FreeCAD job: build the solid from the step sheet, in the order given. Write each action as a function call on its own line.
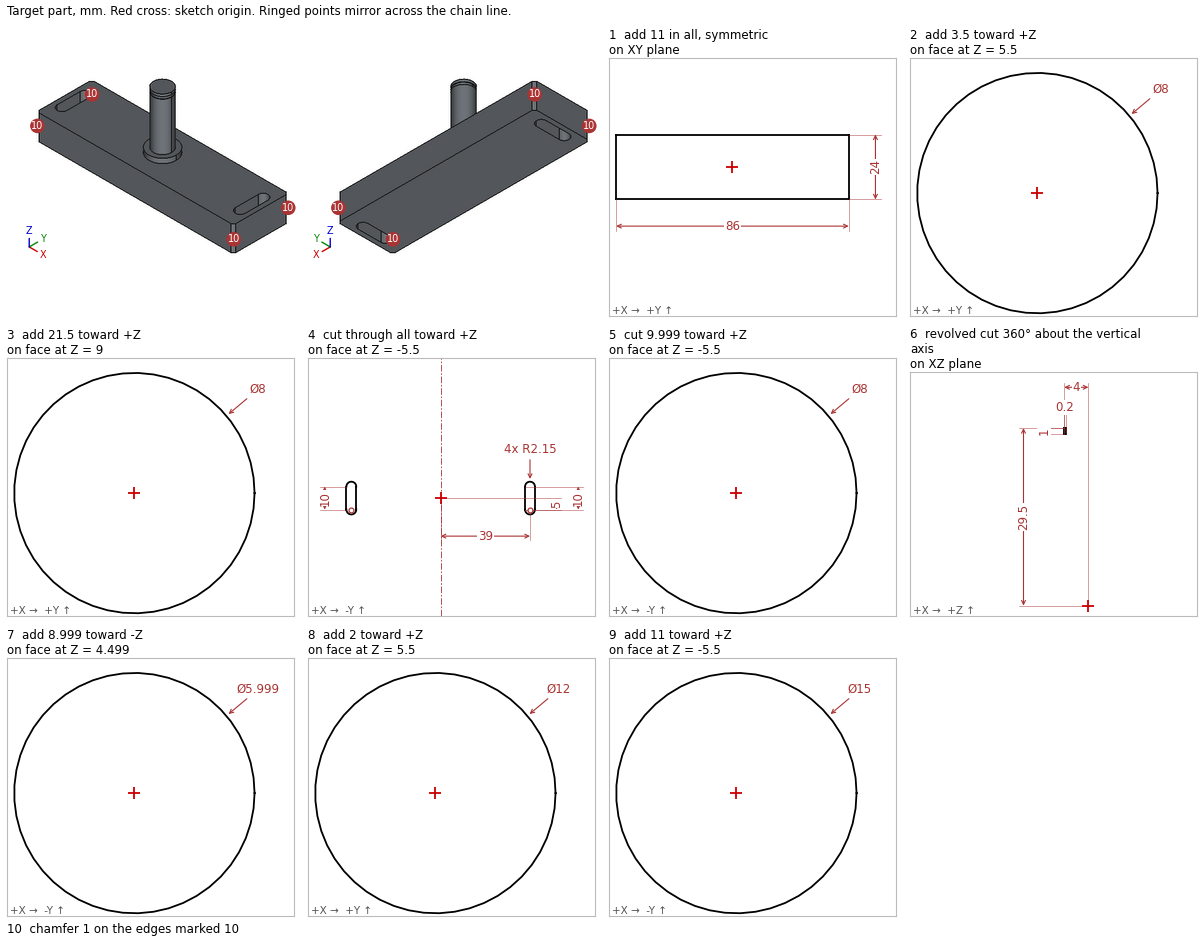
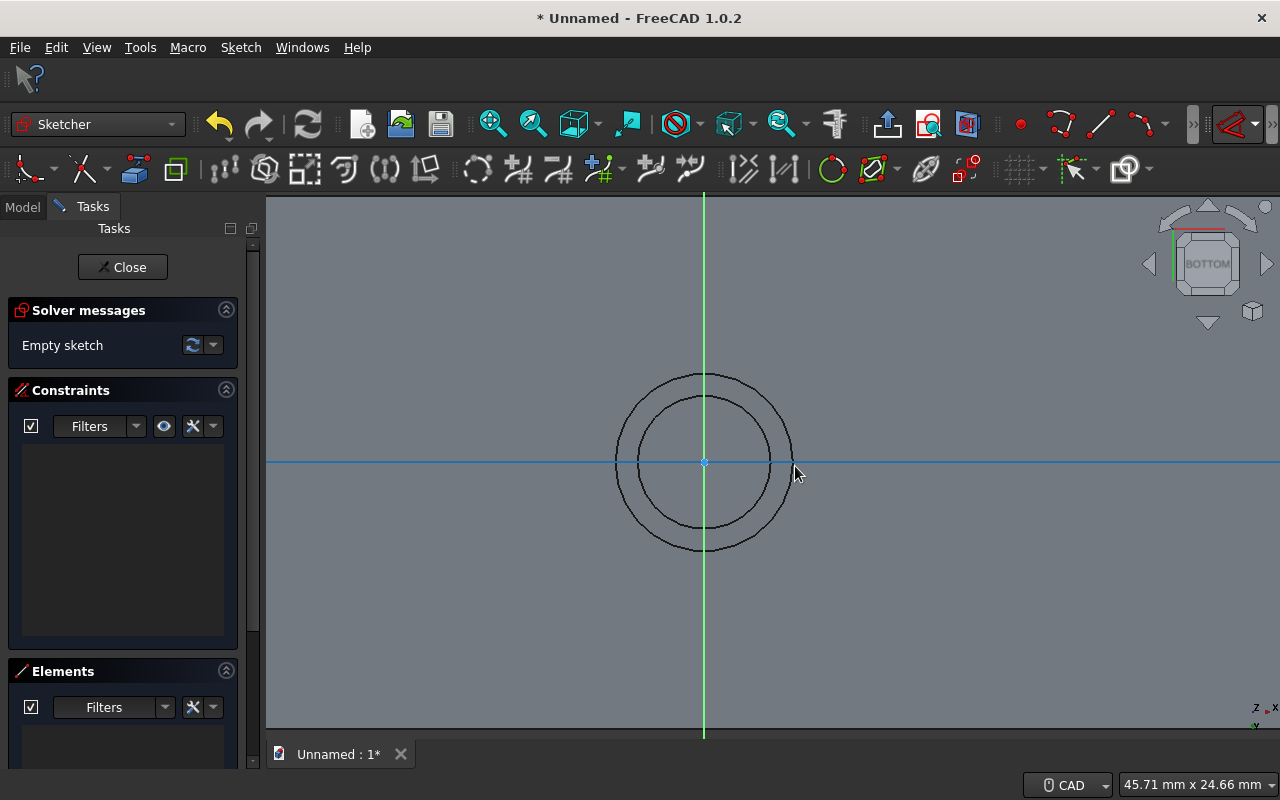
key(g)
key(c)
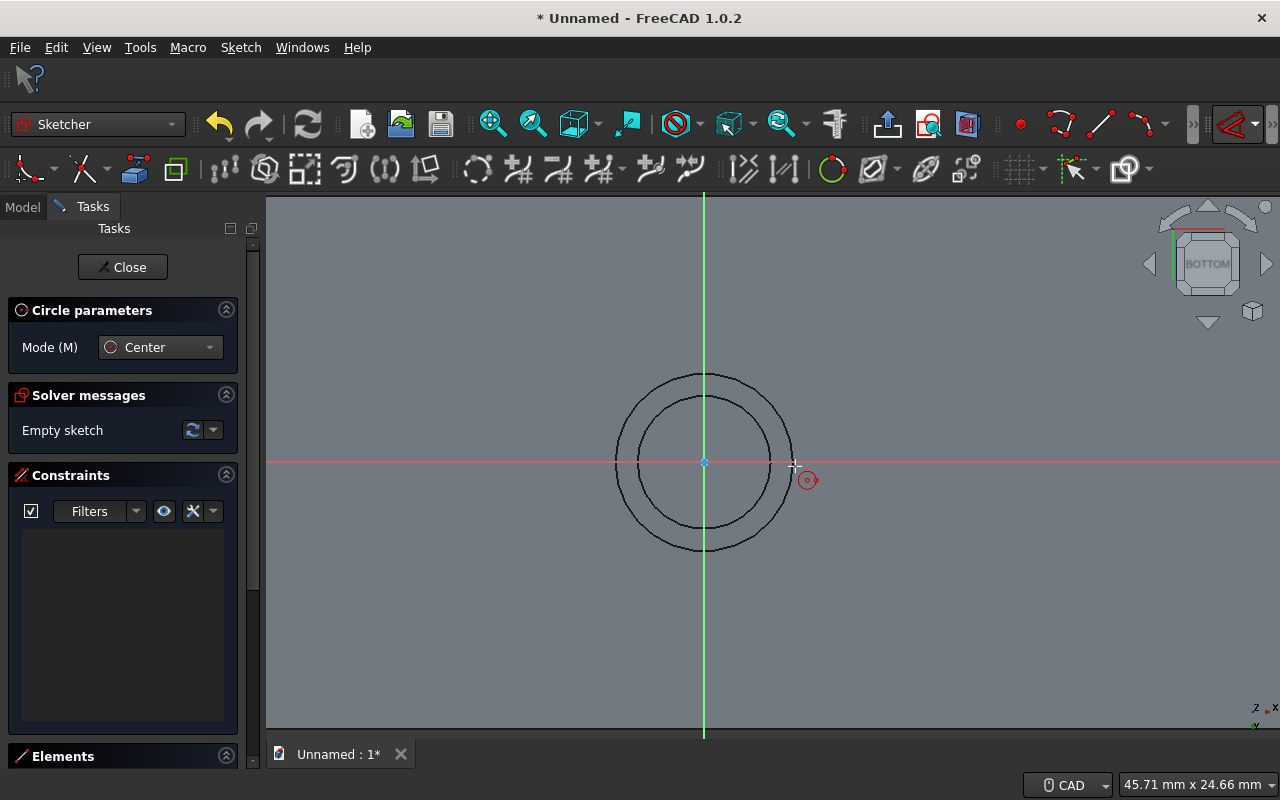
click(704, 462)
move(822, 345)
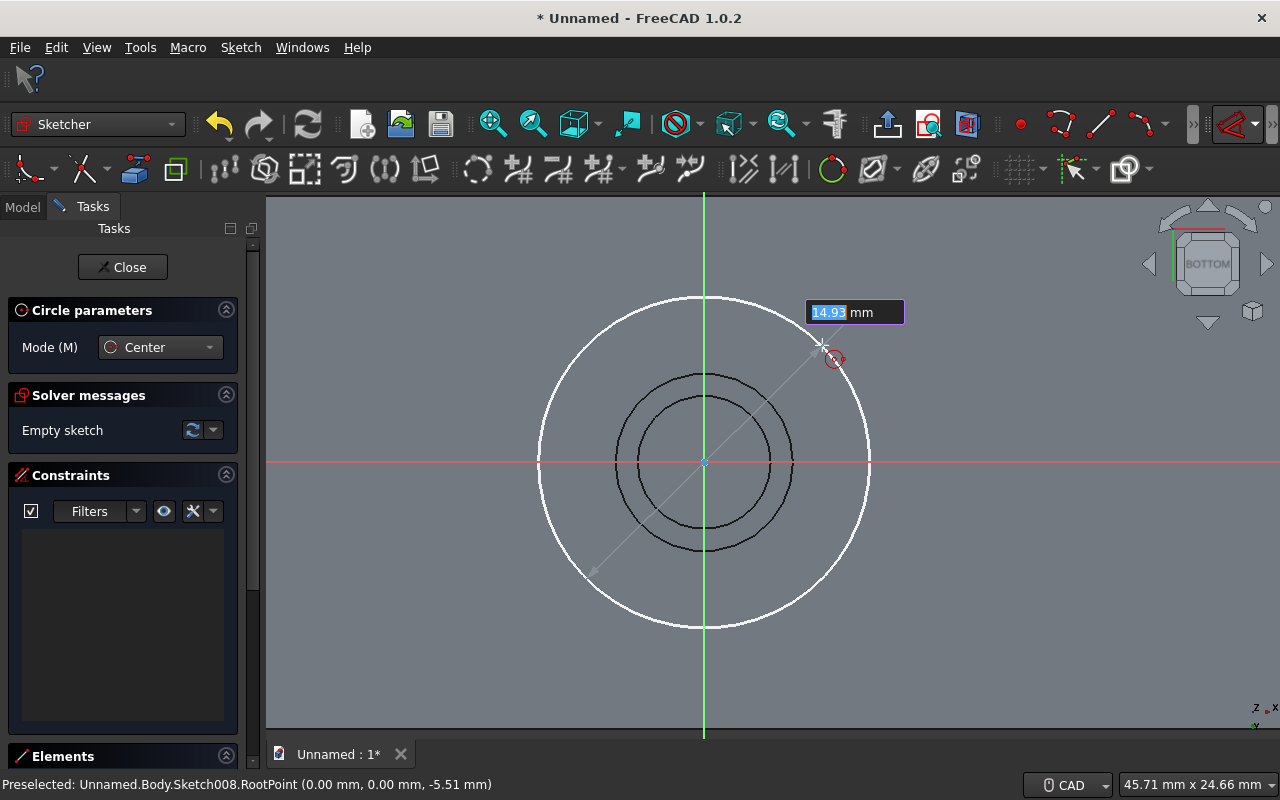
text(15)
key(Return)
key(Escape)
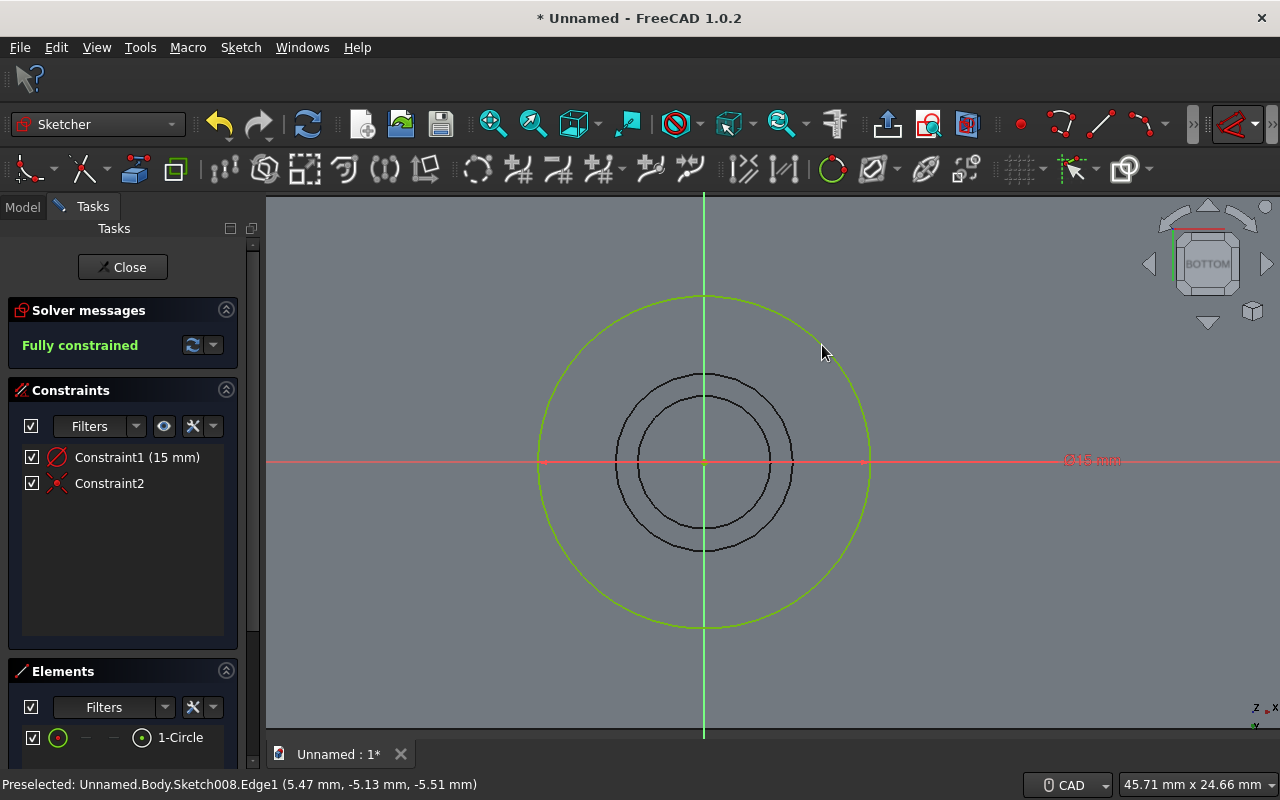
click(123, 267)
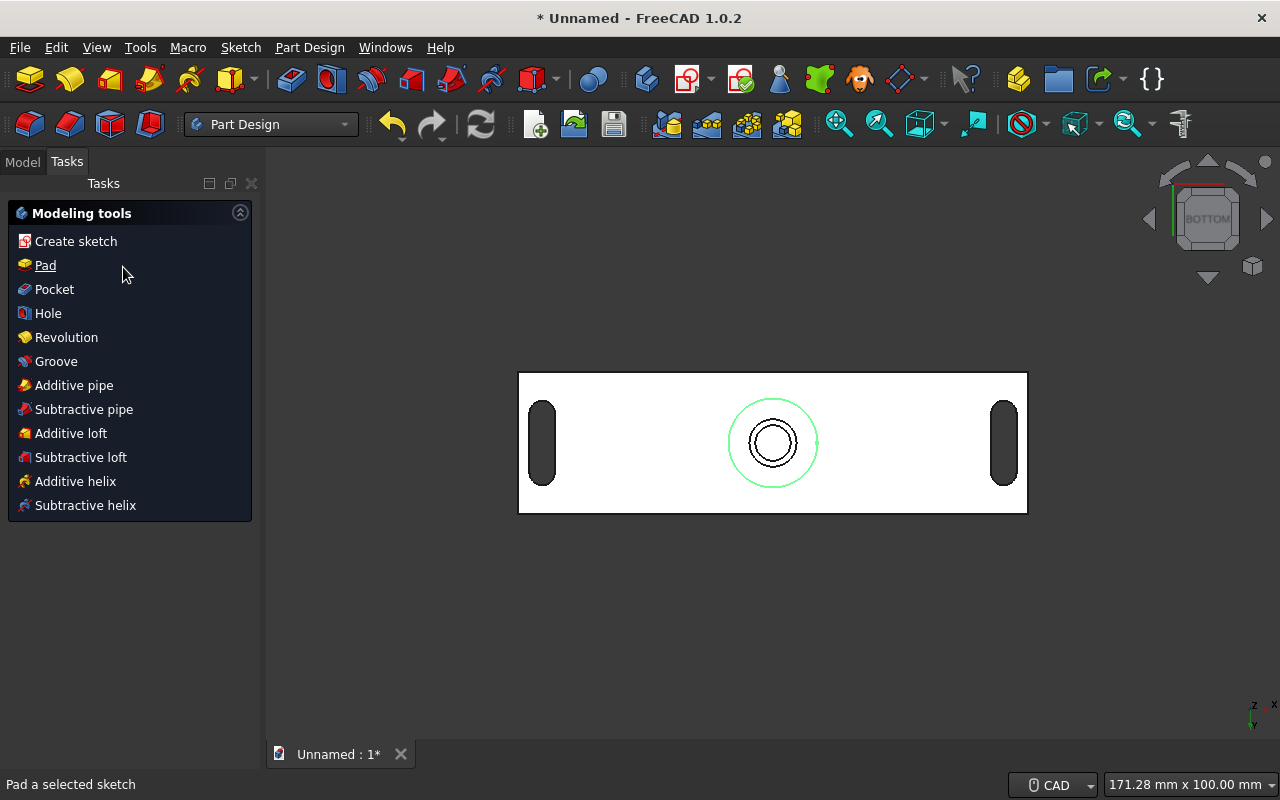
click(30, 80)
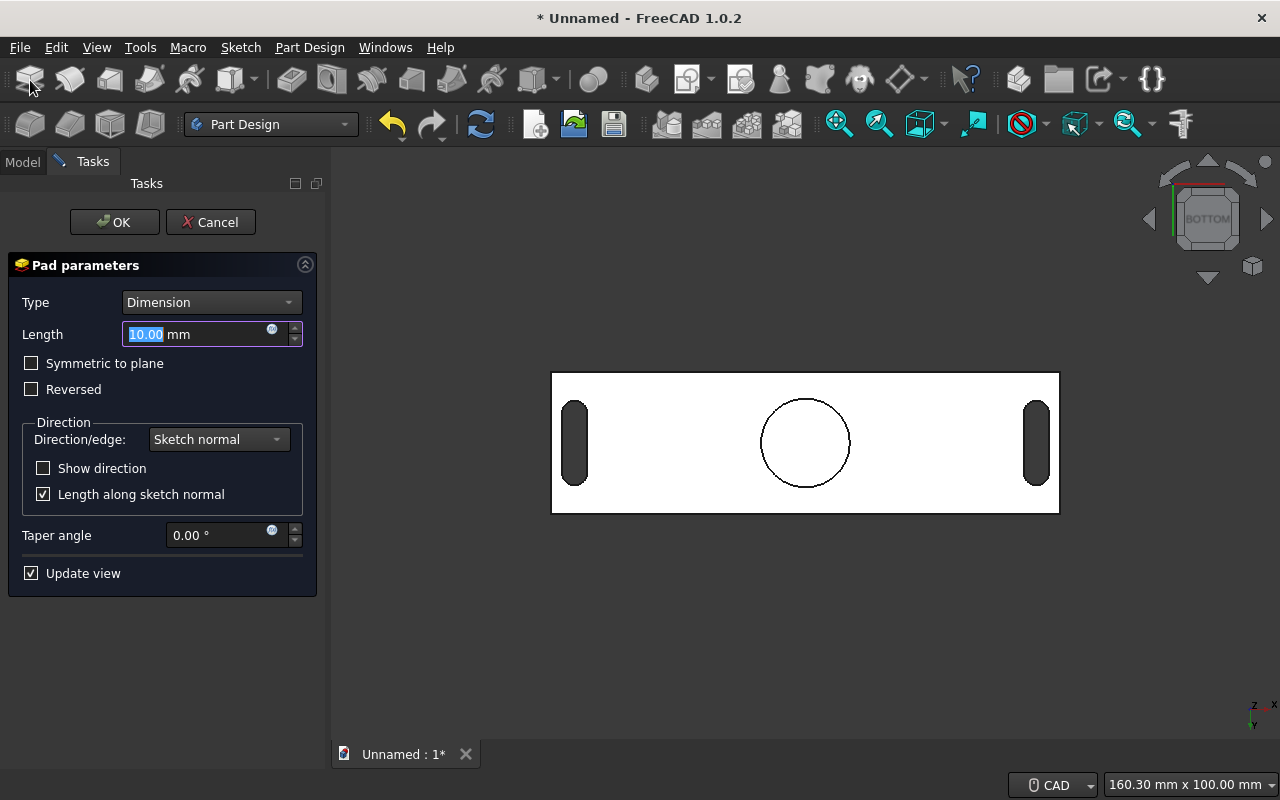
text(11)
key(Tab)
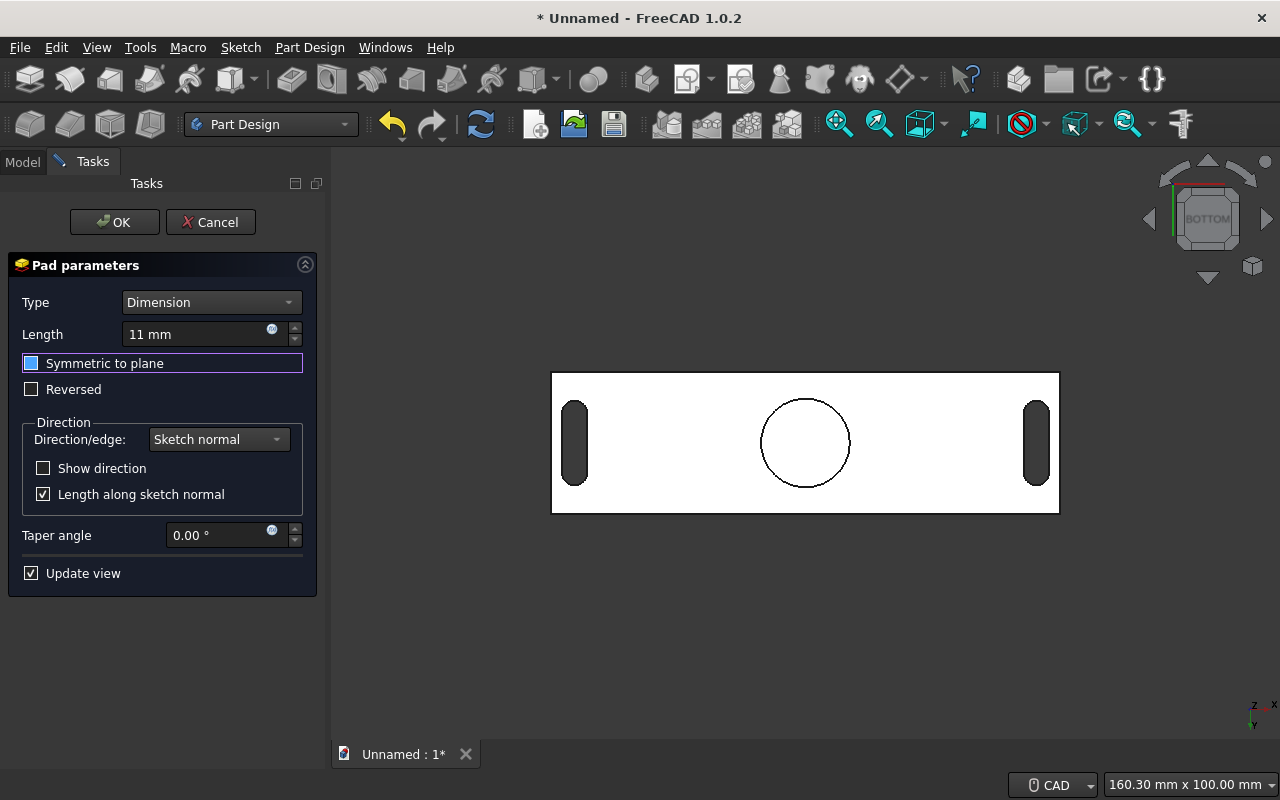
click(30, 389)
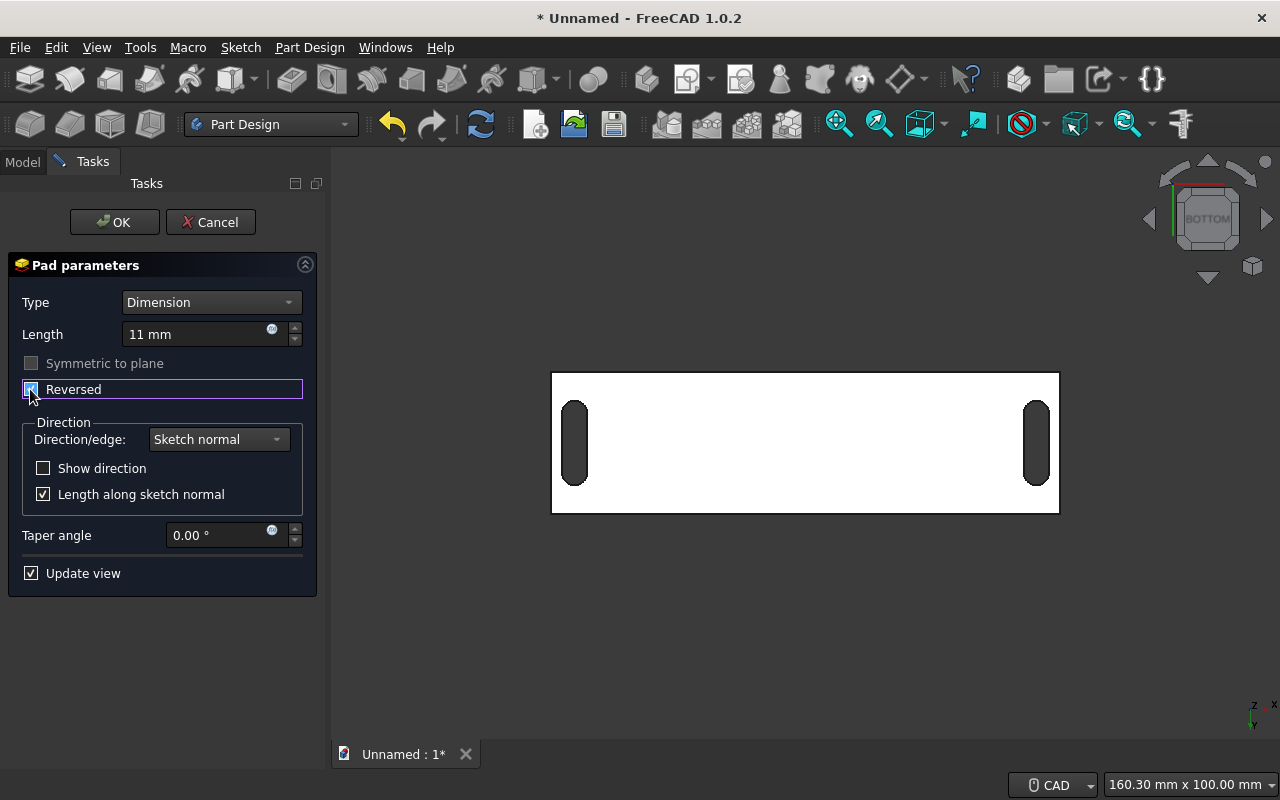
click(115, 222)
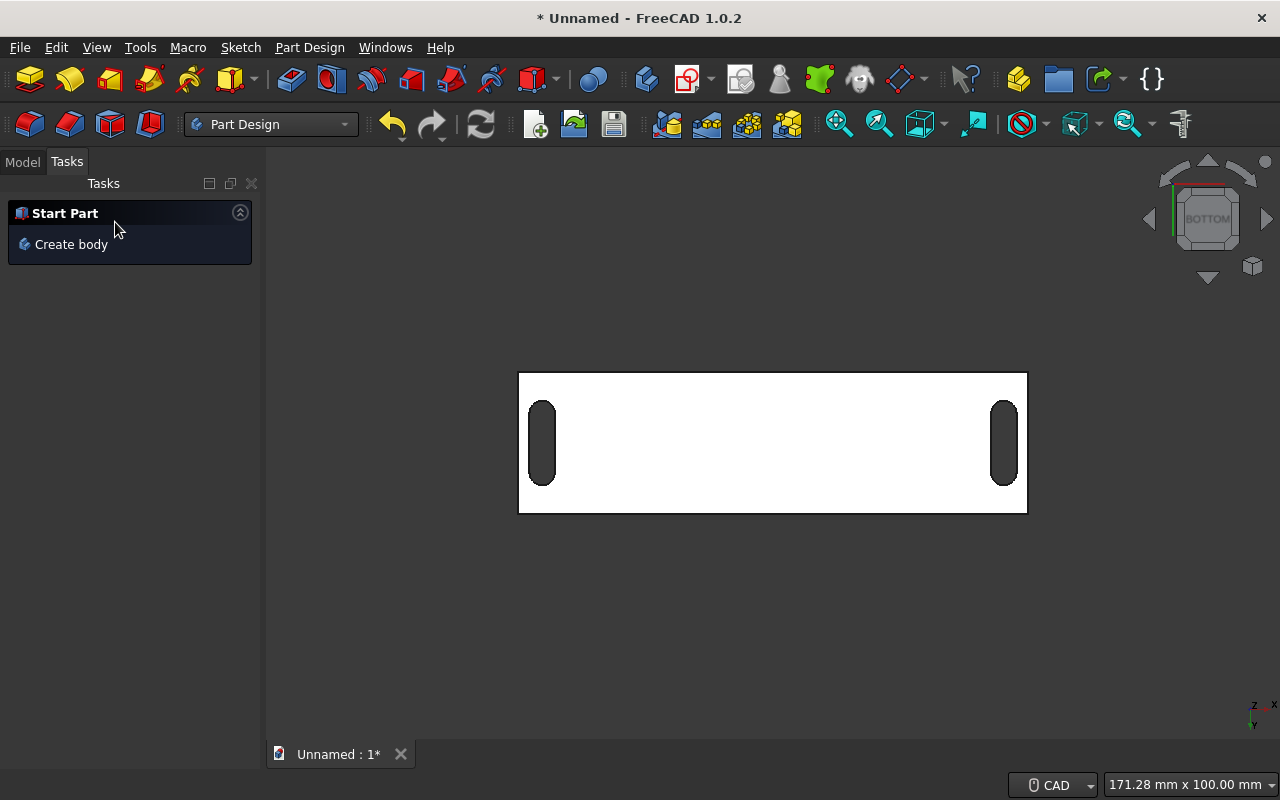
key(0)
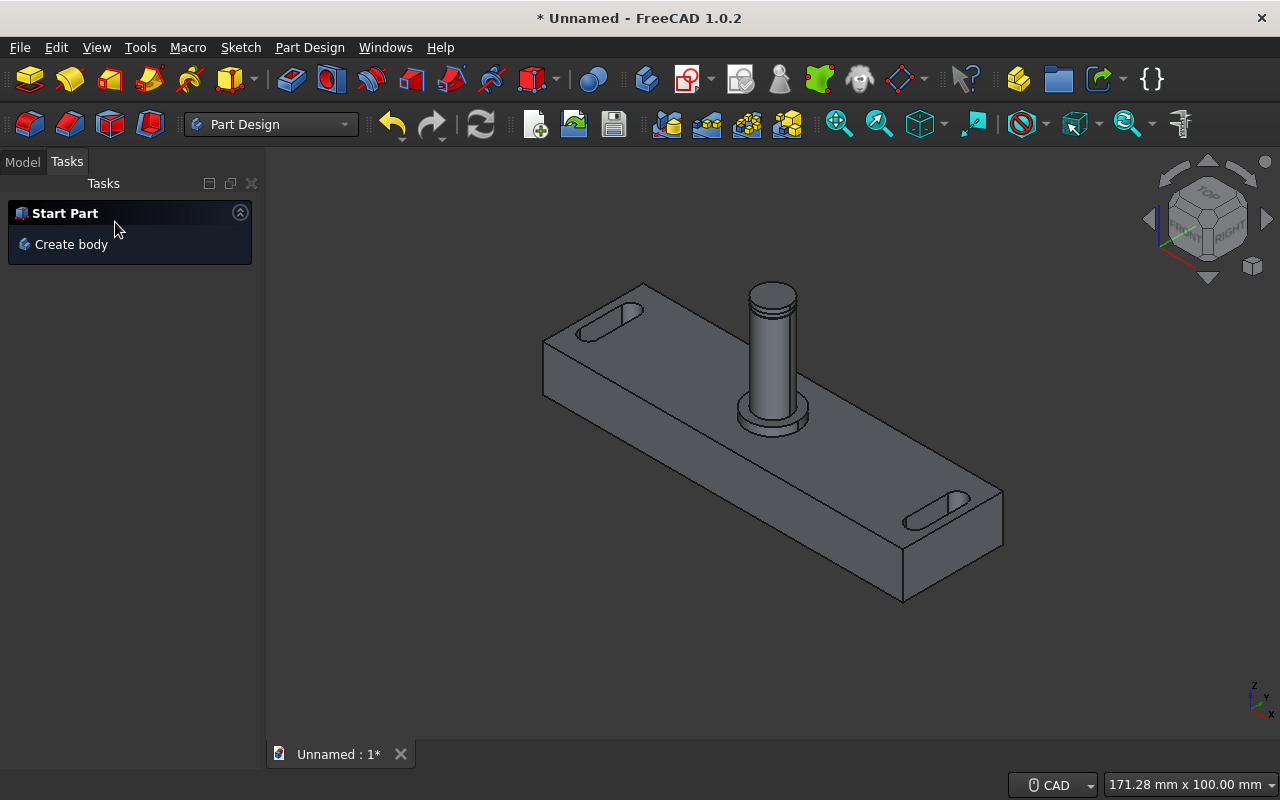
click(903, 575)